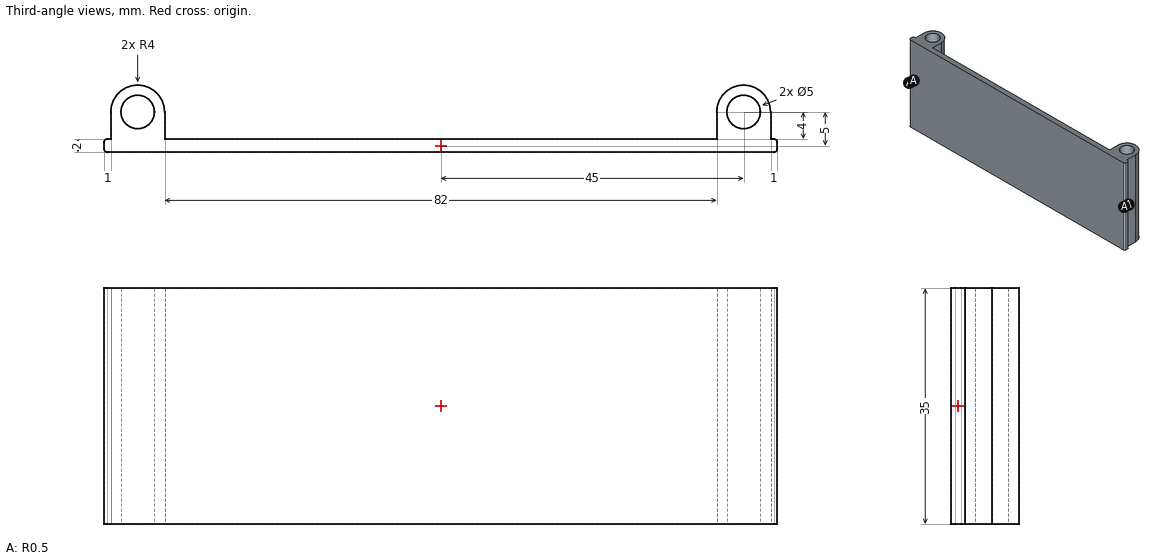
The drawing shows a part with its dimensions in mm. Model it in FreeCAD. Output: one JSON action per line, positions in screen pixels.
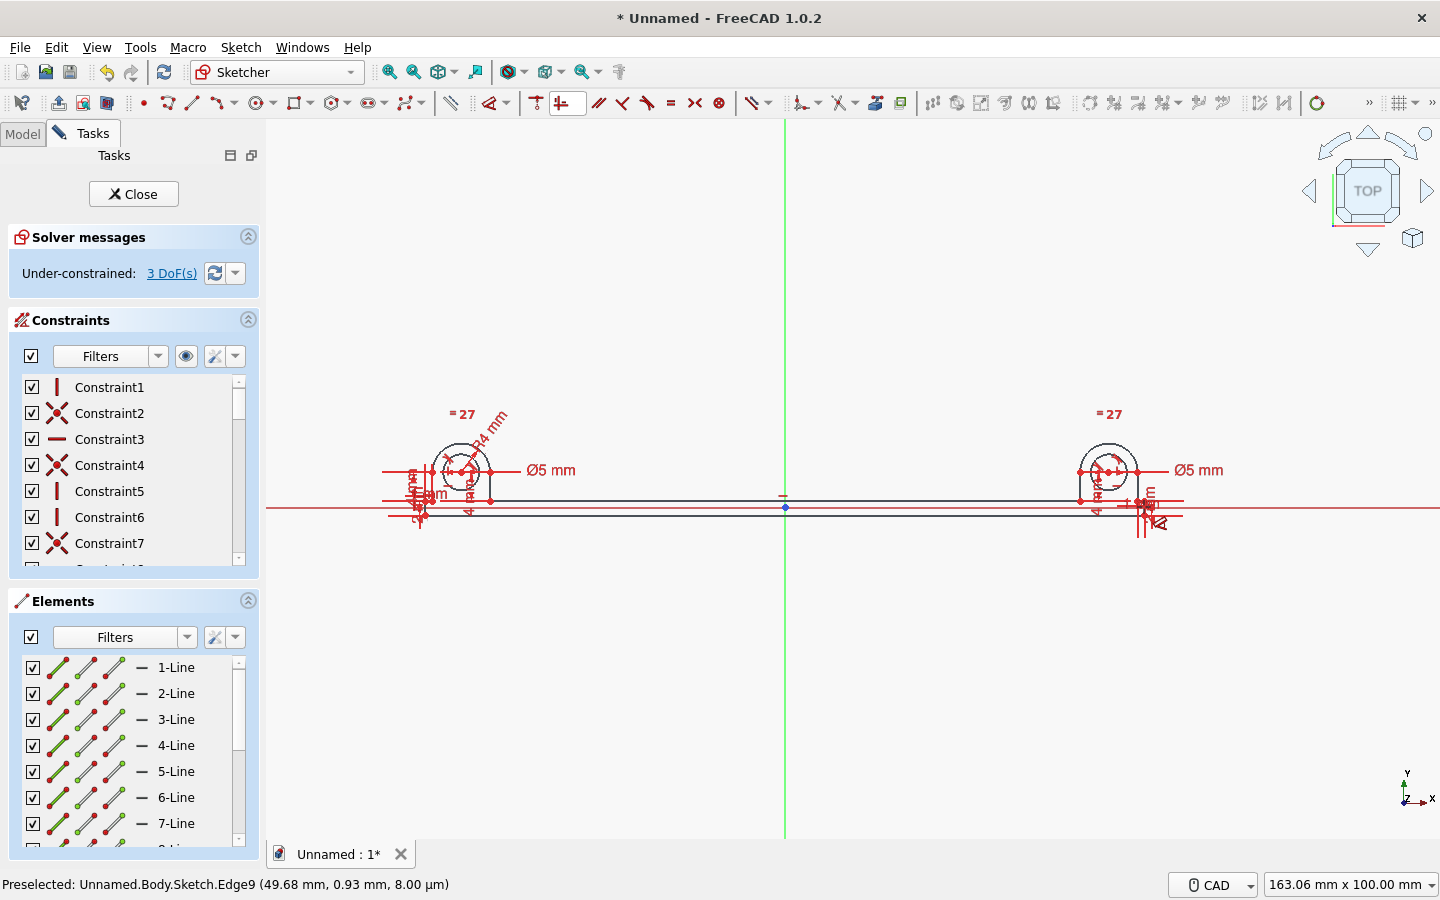
{"action": "left_click", "coordinate": [1109, 472]}
{"action": "left_click", "coordinate": [751, 482]}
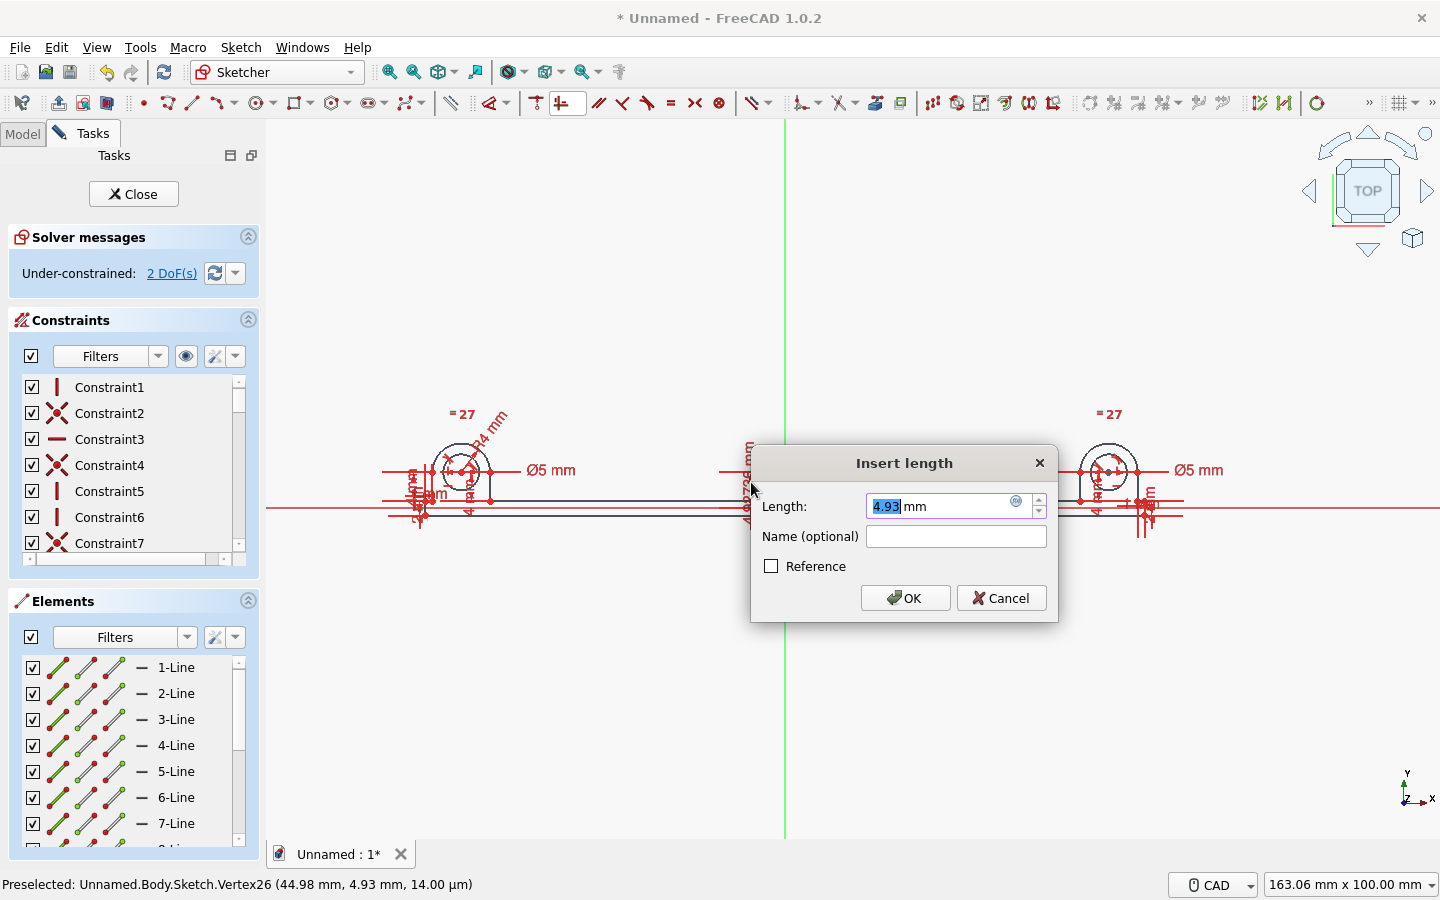
{"action": "type", "text": "5"}
{"action": "key", "text": "Return"}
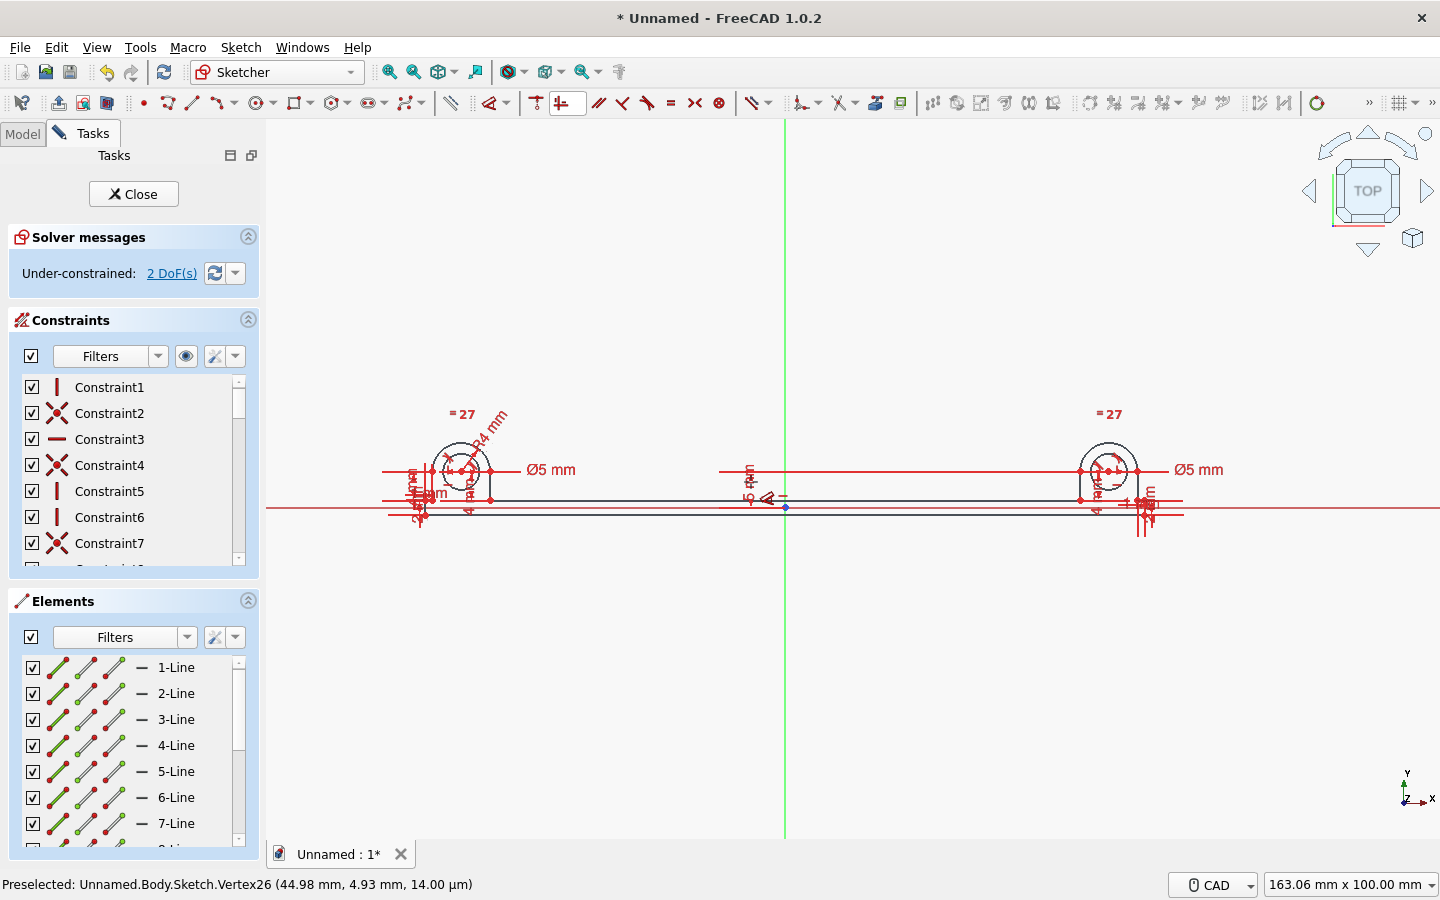
{"action": "scroll", "coordinate": [903, 501], "scroll_direction": "up", "scroll_amount": 4}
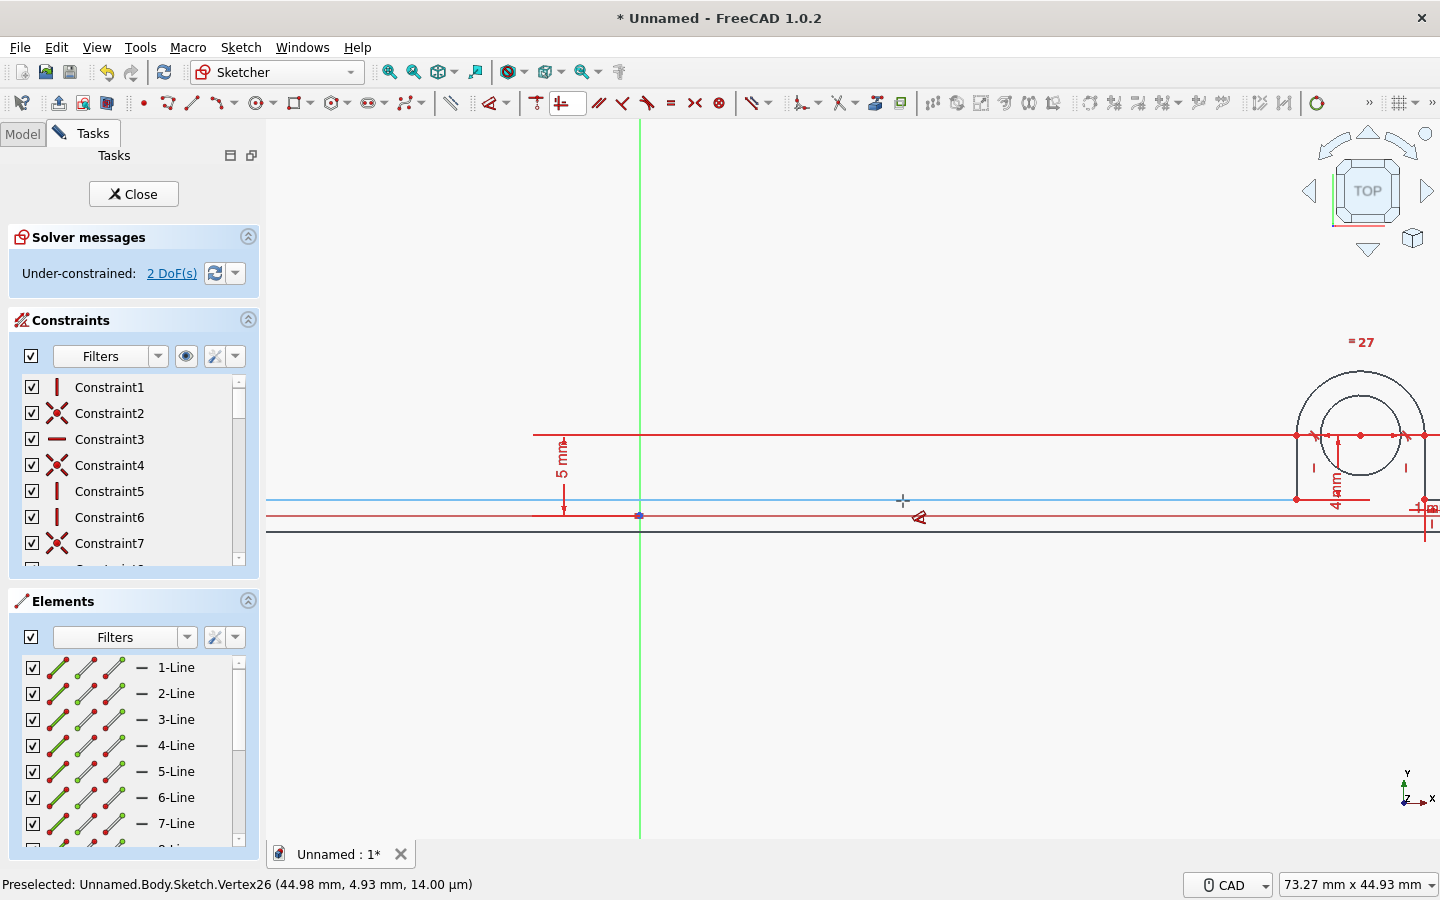
{"action": "left_click", "coordinate": [903, 500]}
{"action": "left_click", "coordinate": [784, 466]}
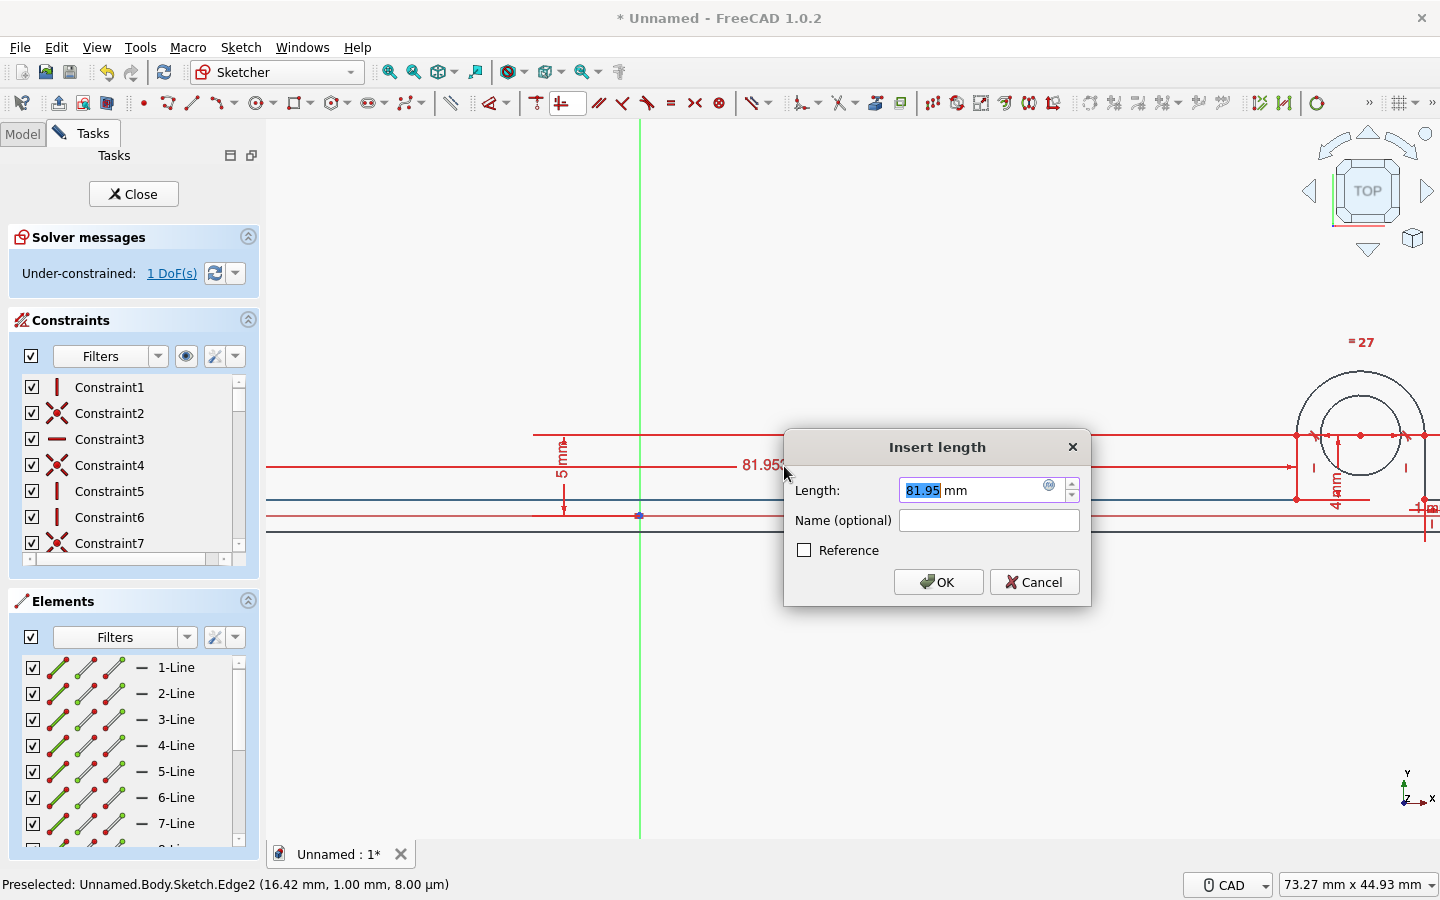
{"action": "type", "text": "82"}
{"action": "key", "text": "Return"}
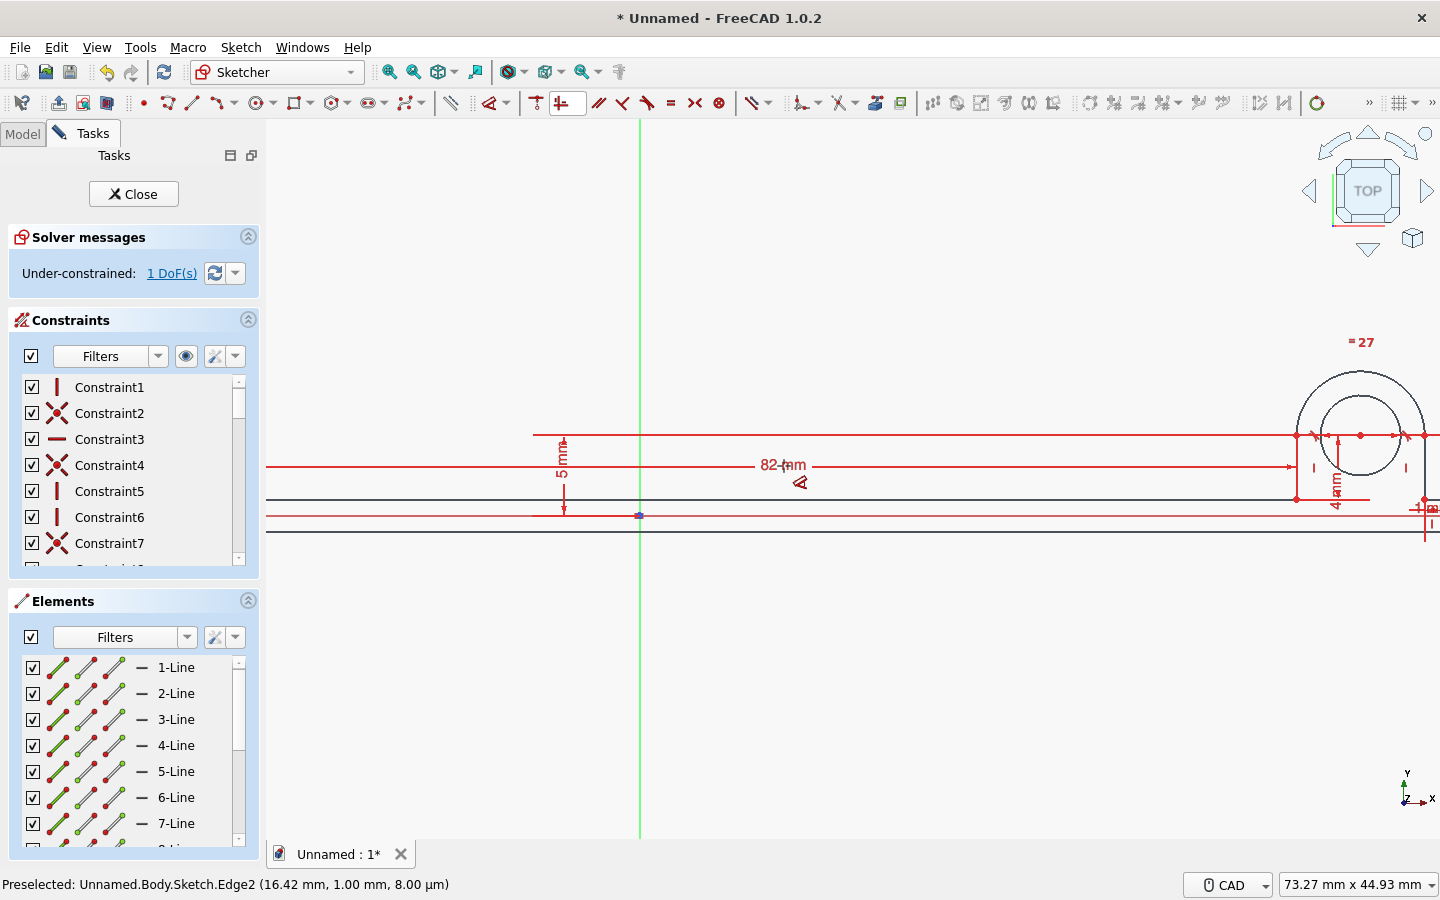
{"action": "scroll", "coordinate": [903, 501], "scroll_direction": "down", "scroll_amount": 4}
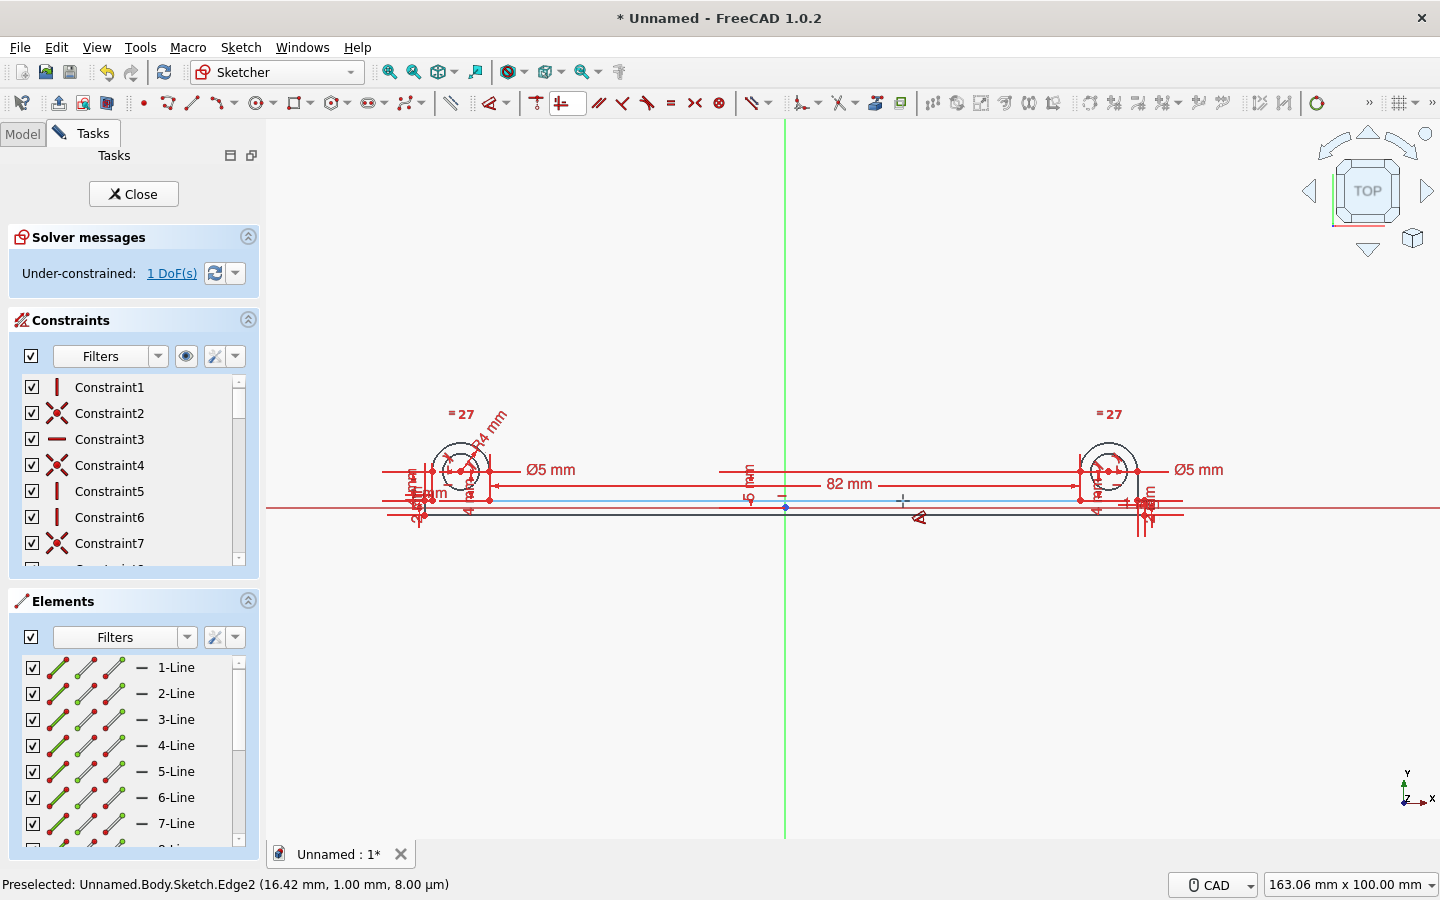
{"action": "left_click", "coordinate": [1109, 472]}
{"action": "left_click", "coordinate": [947, 542]}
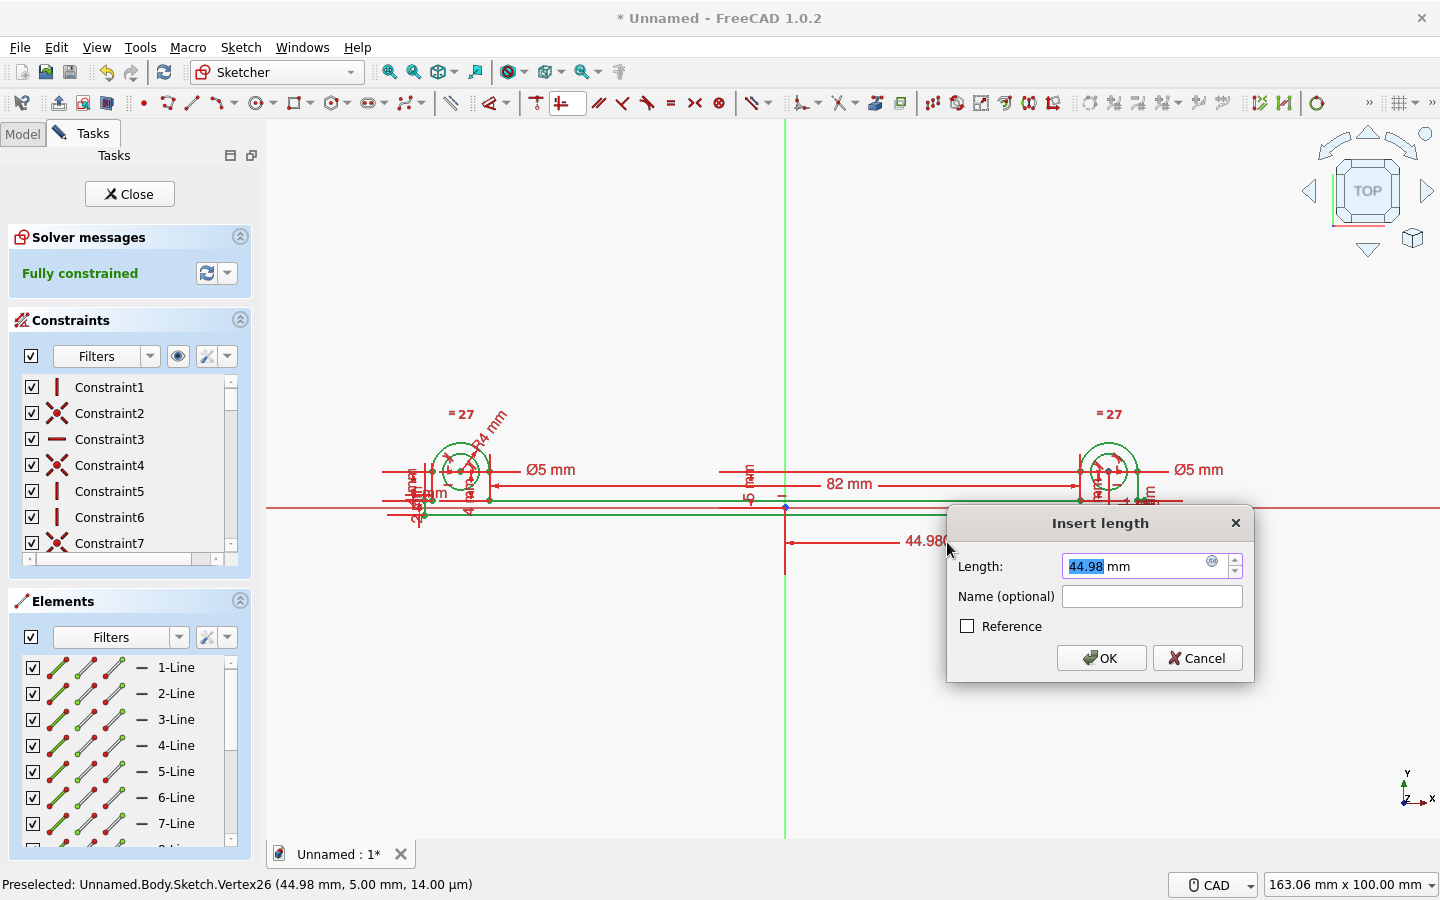
{"action": "type", "text": "45"}
{"action": "key", "text": "Return"}
{"action": "key", "text": "Escape"}